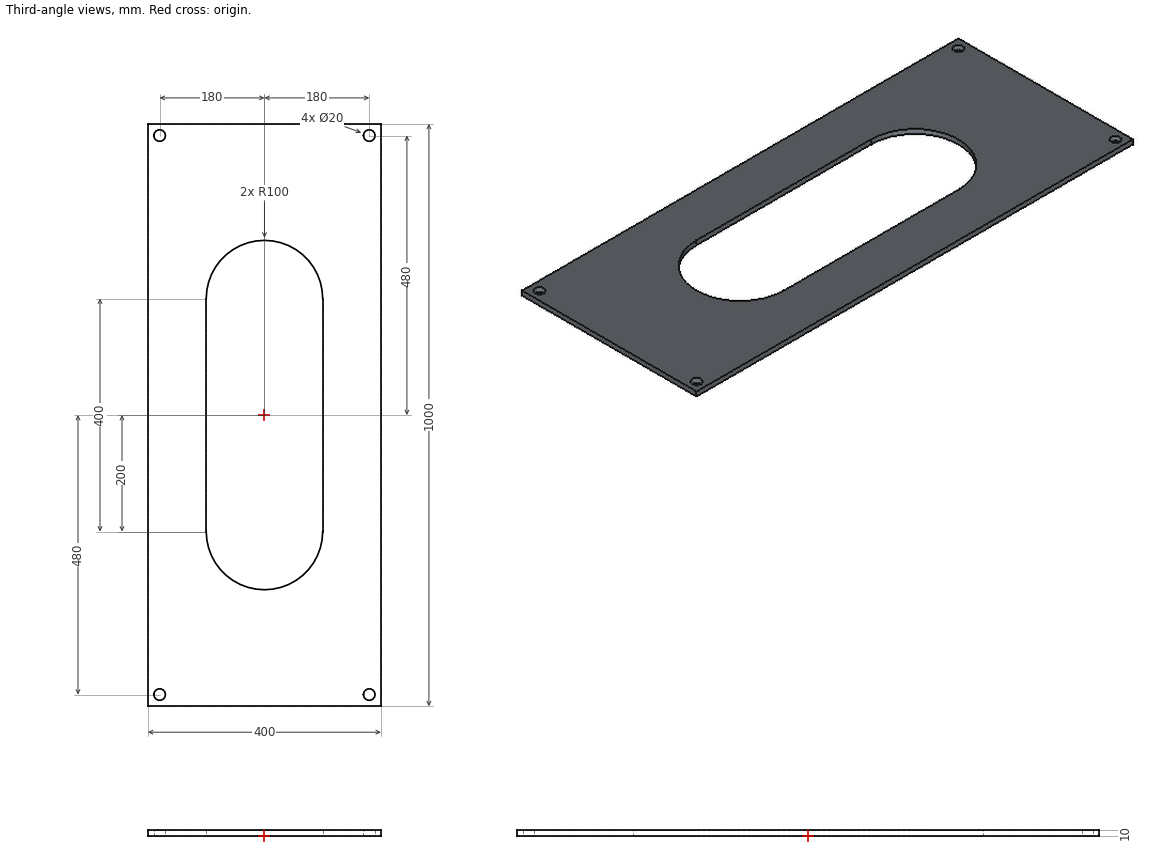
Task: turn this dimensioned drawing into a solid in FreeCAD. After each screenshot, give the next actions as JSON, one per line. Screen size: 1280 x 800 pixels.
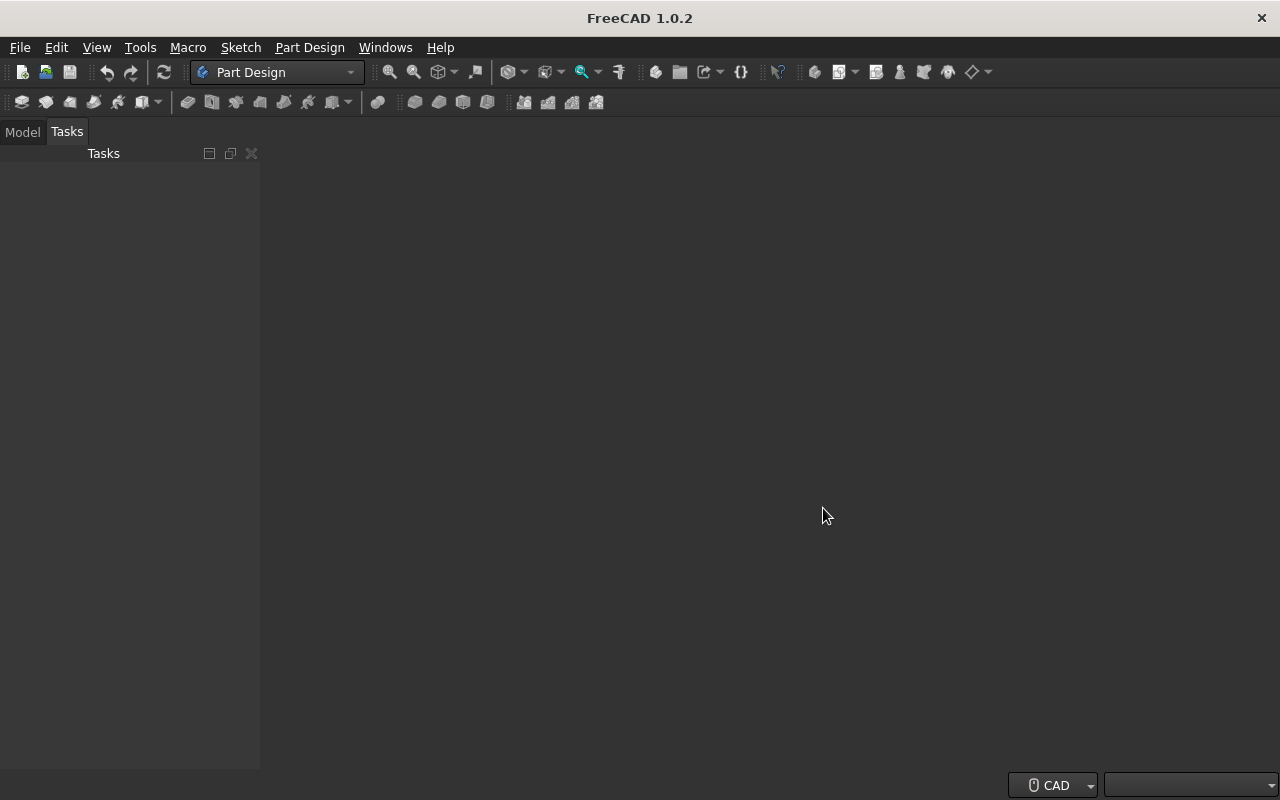
{"action": "left_click", "coordinate": [22, 72]}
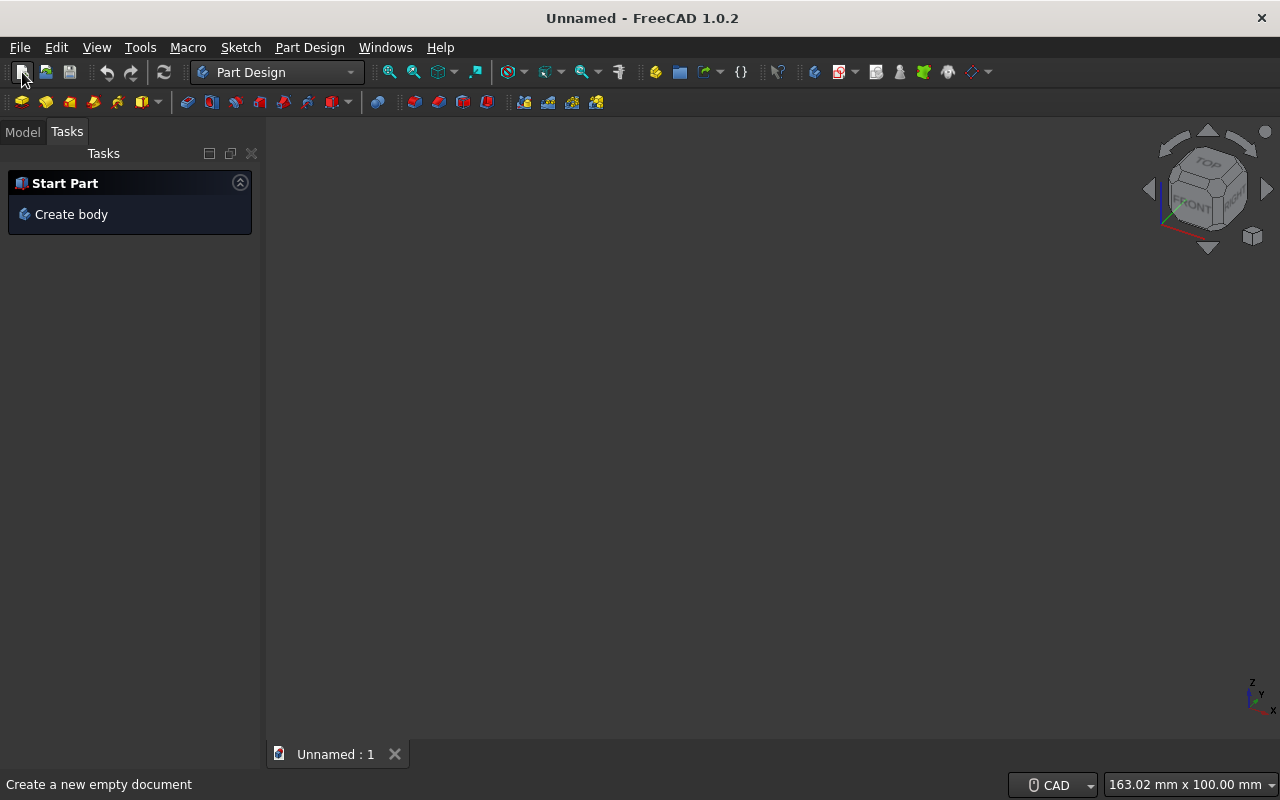
{"action": "left_click", "coordinate": [840, 72]}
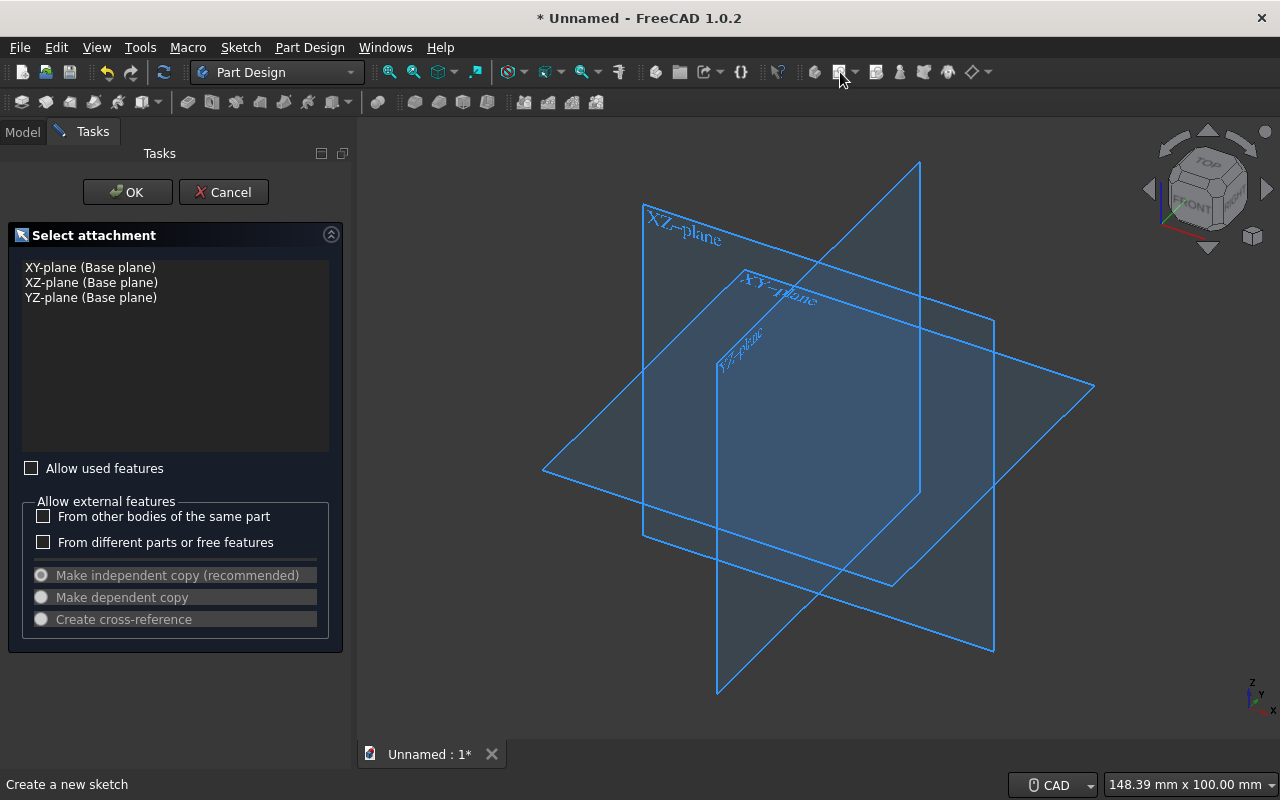
{"action": "left_click", "coordinate": [82, 268]}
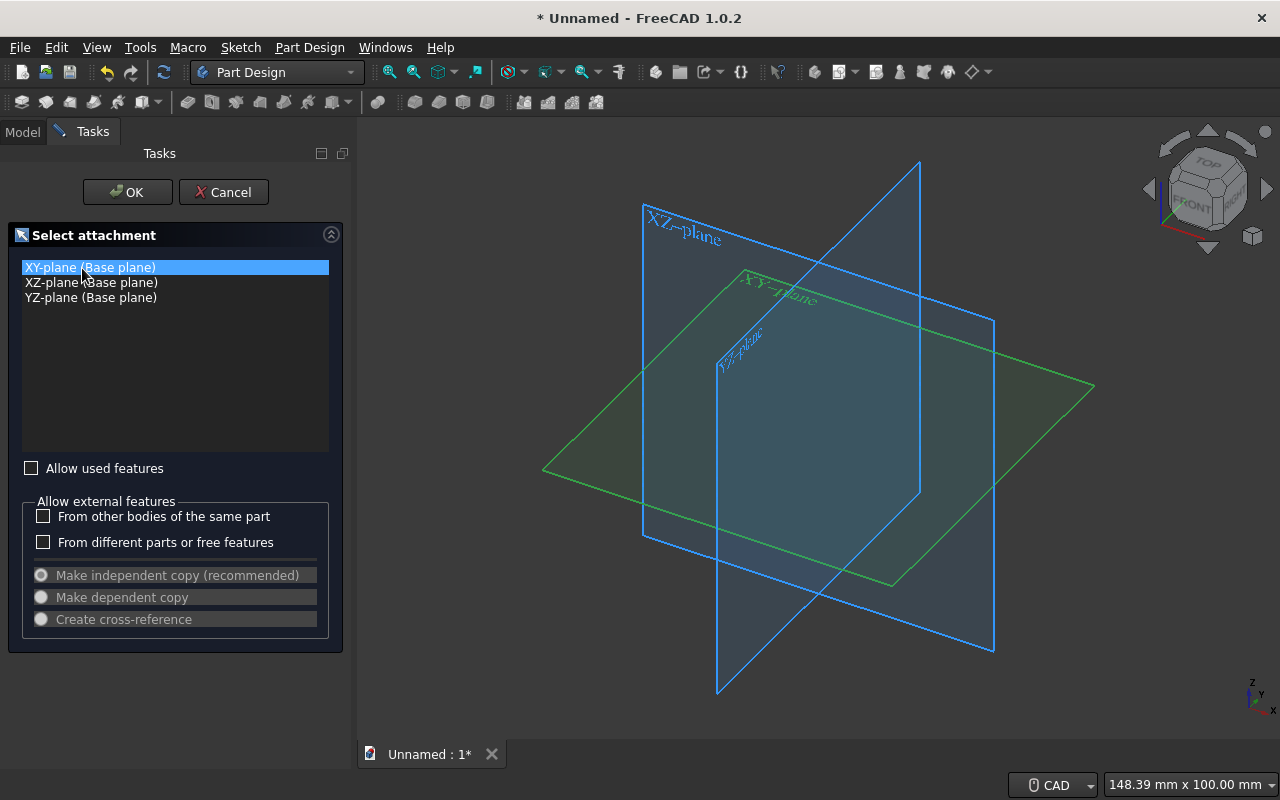
{"action": "left_click", "coordinate": [128, 192]}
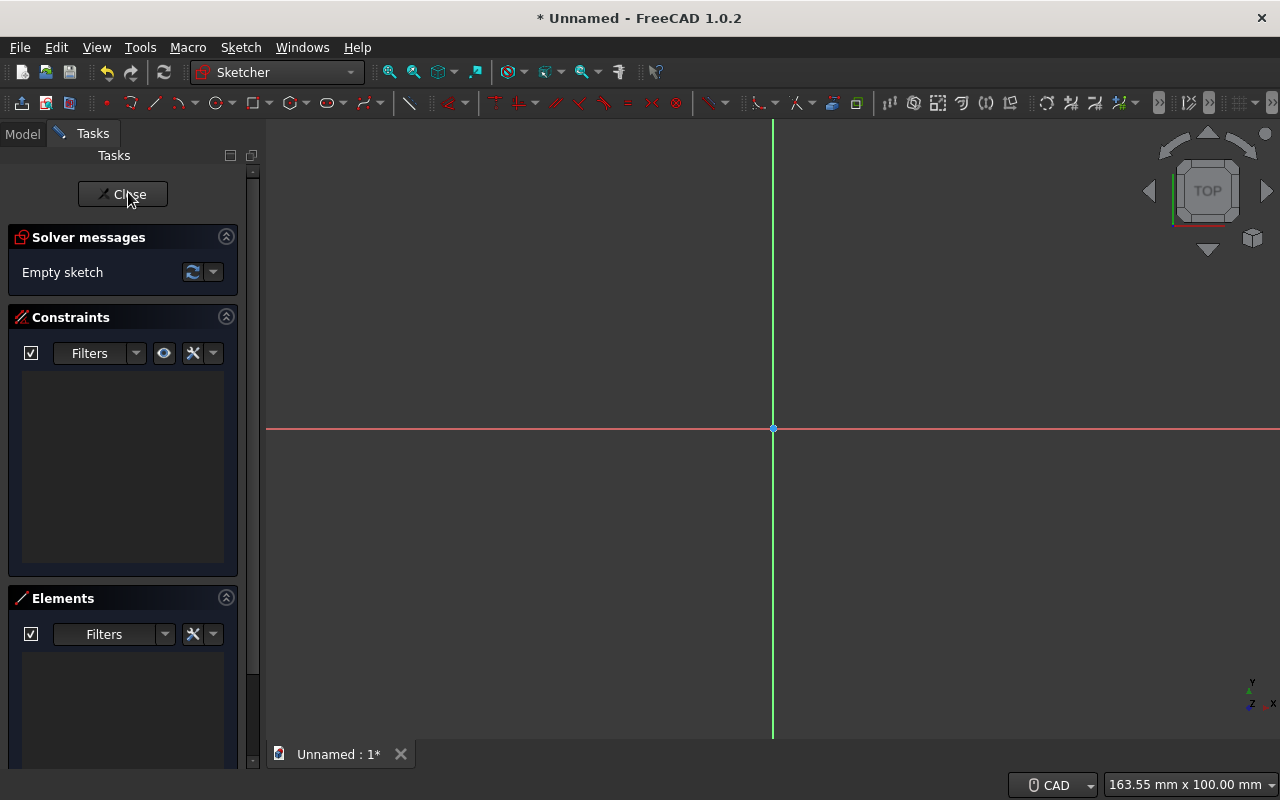
{"action": "scroll", "coordinate": [700, 429], "scroll_direction": "down", "scroll_amount": 14}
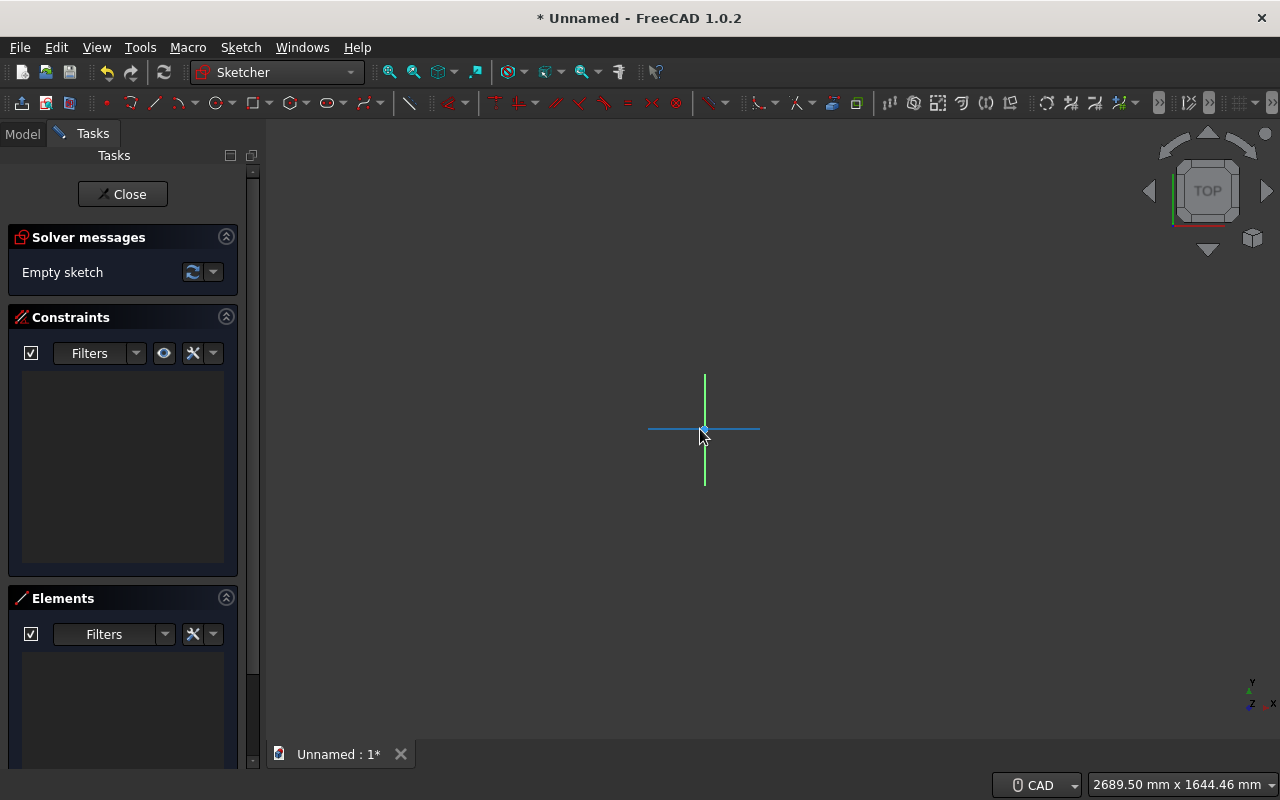
{"action": "left_click", "coordinate": [272, 104]}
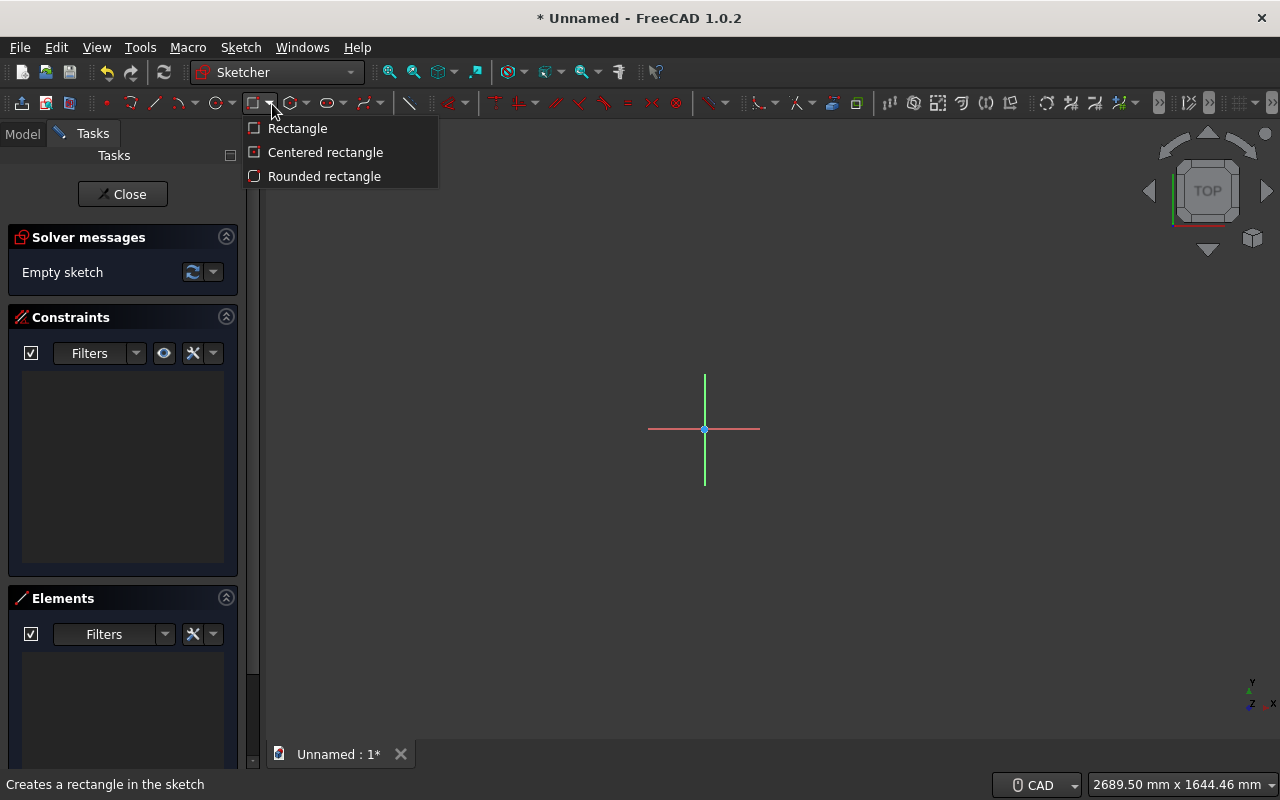
{"action": "left_click", "coordinate": [340, 152]}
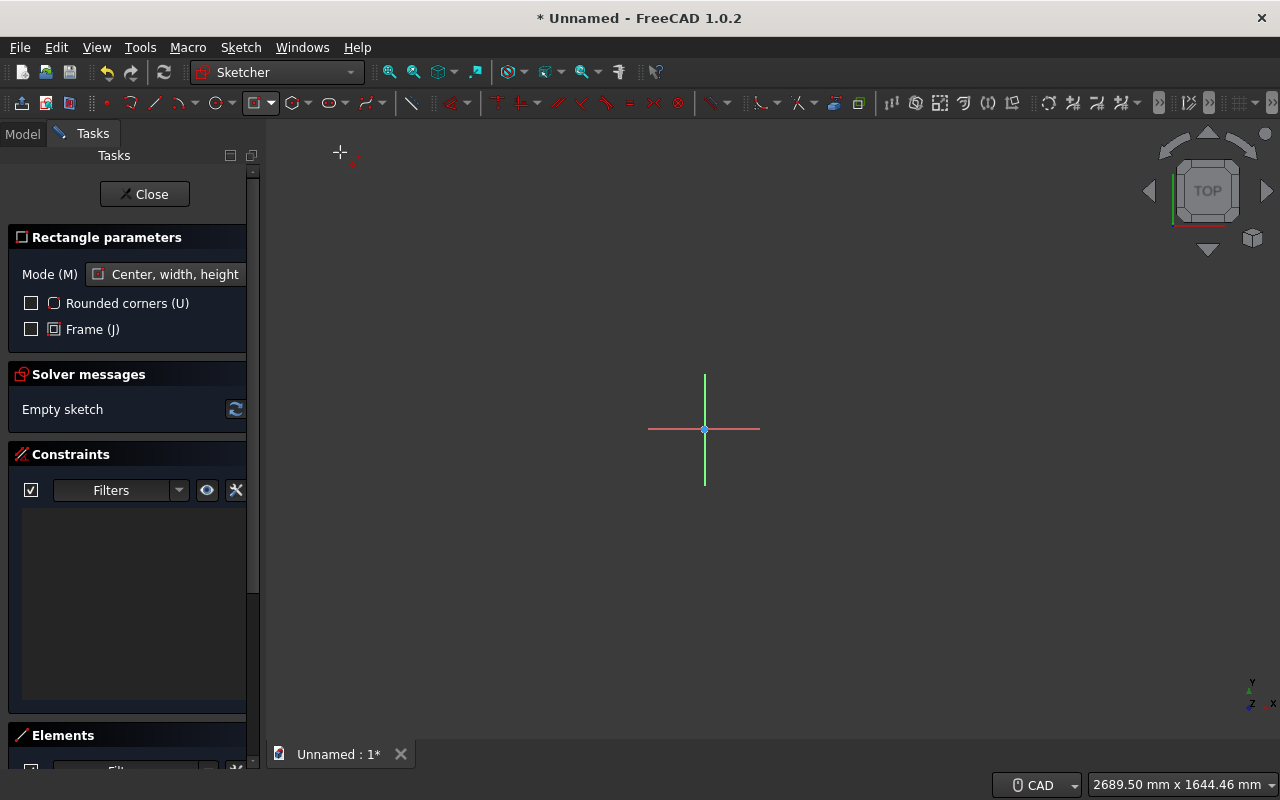
{"action": "left_click", "coordinate": [705, 429]}
{"action": "mouse_move", "coordinate": [780, 241]}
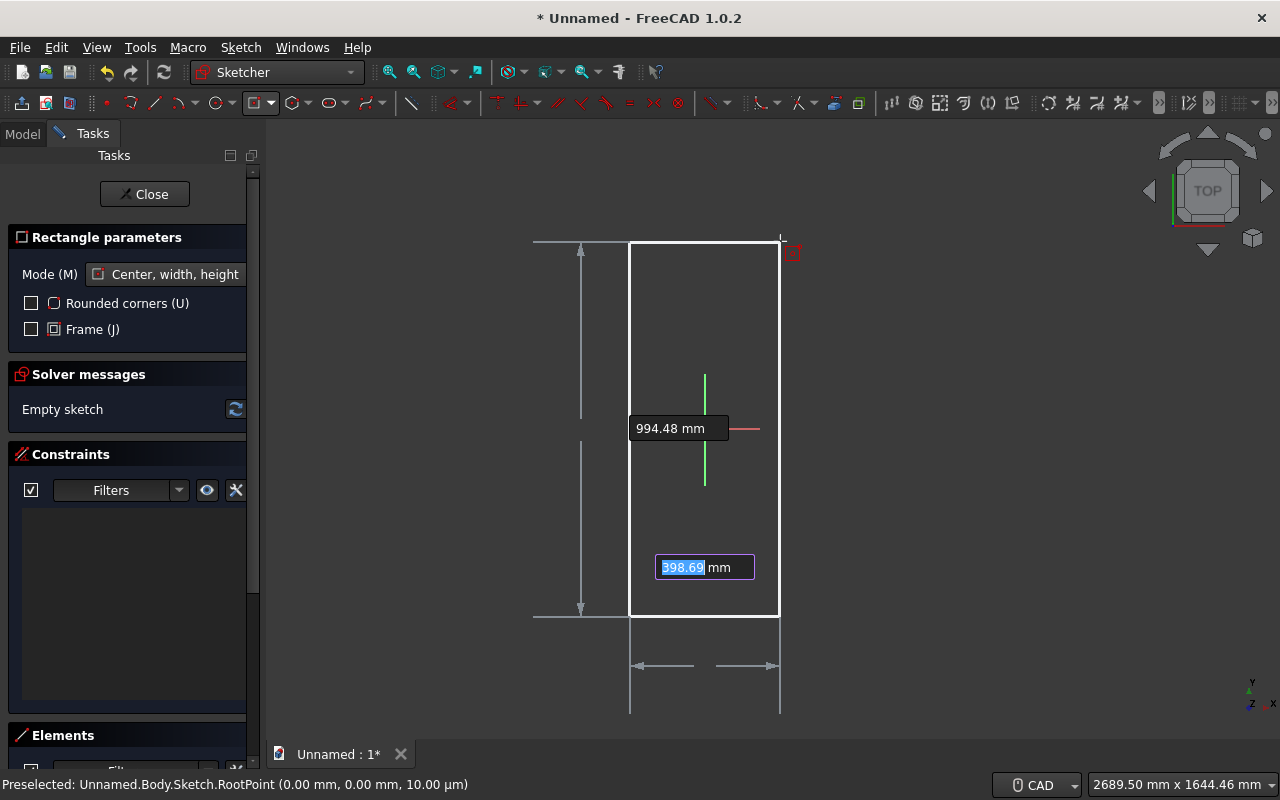
{"action": "type", "text": "400"}
{"action": "key", "text": "Tab"}
{"action": "type", "text": "1000"}
{"action": "key", "text": "Return"}
{"action": "key", "text": "Escape"}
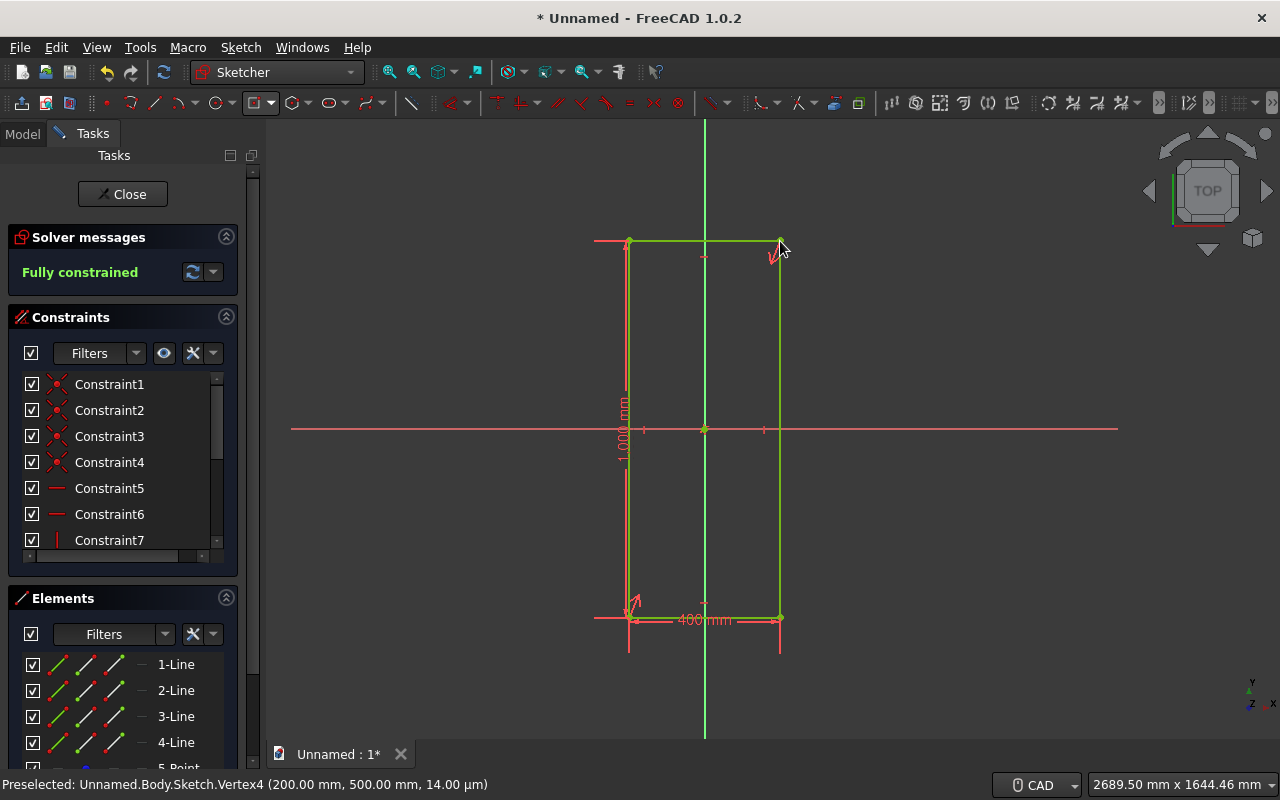
{"action": "left_click", "coordinate": [123, 194]}